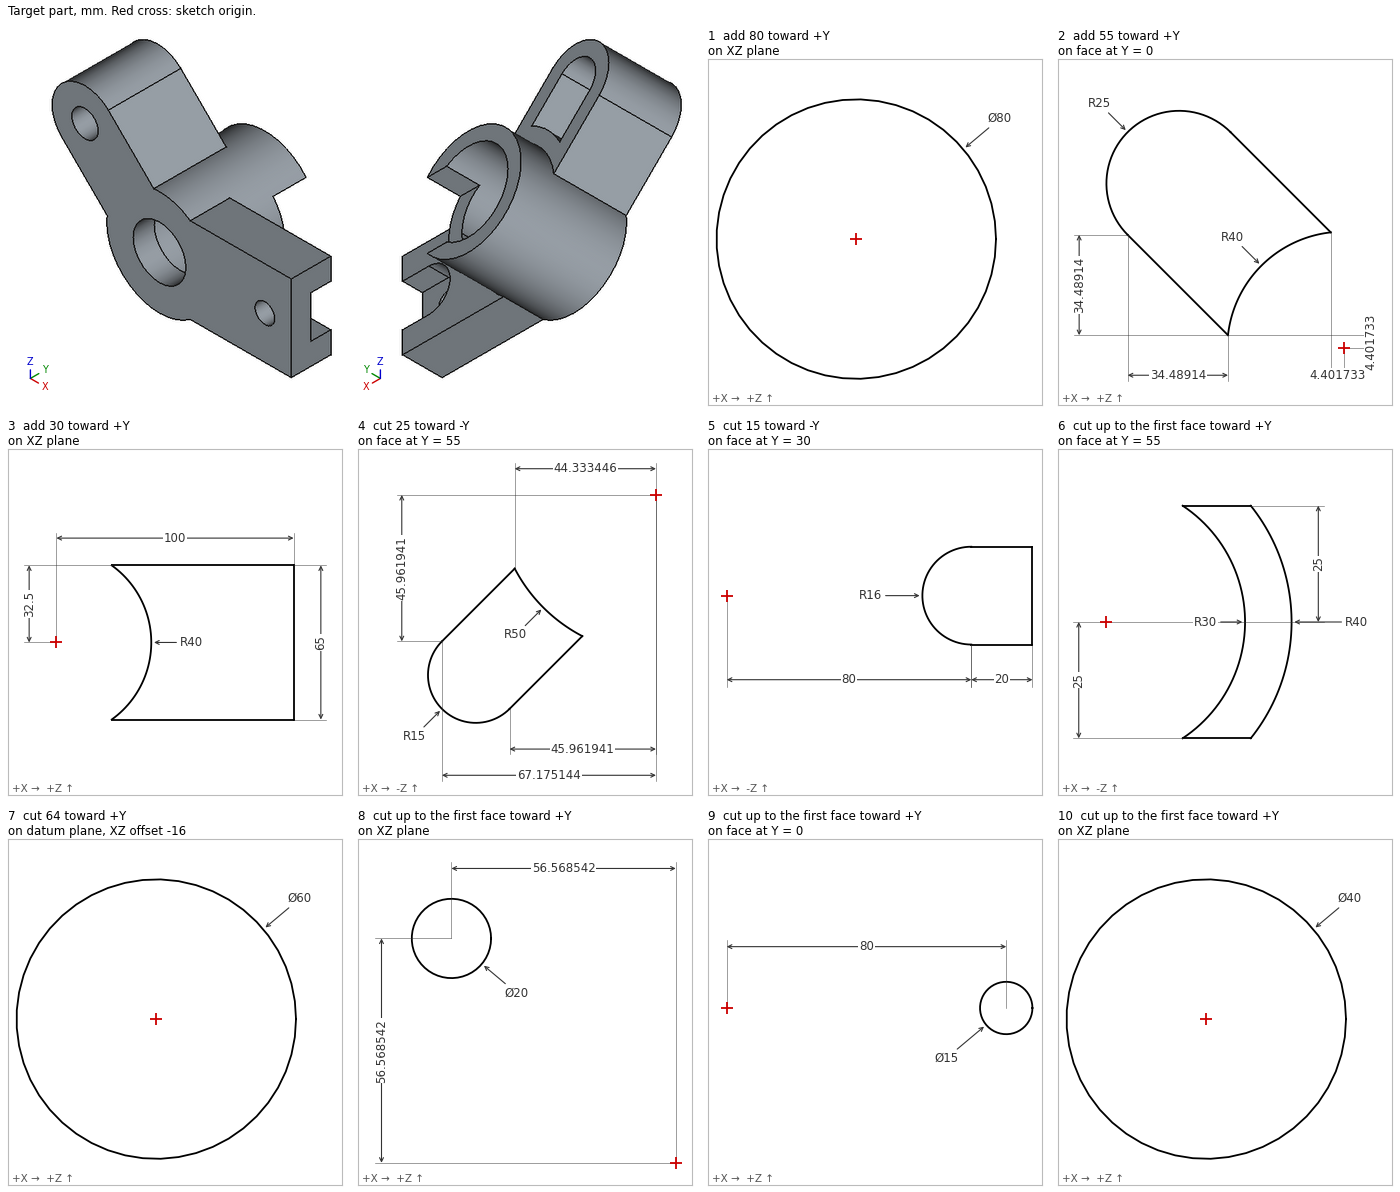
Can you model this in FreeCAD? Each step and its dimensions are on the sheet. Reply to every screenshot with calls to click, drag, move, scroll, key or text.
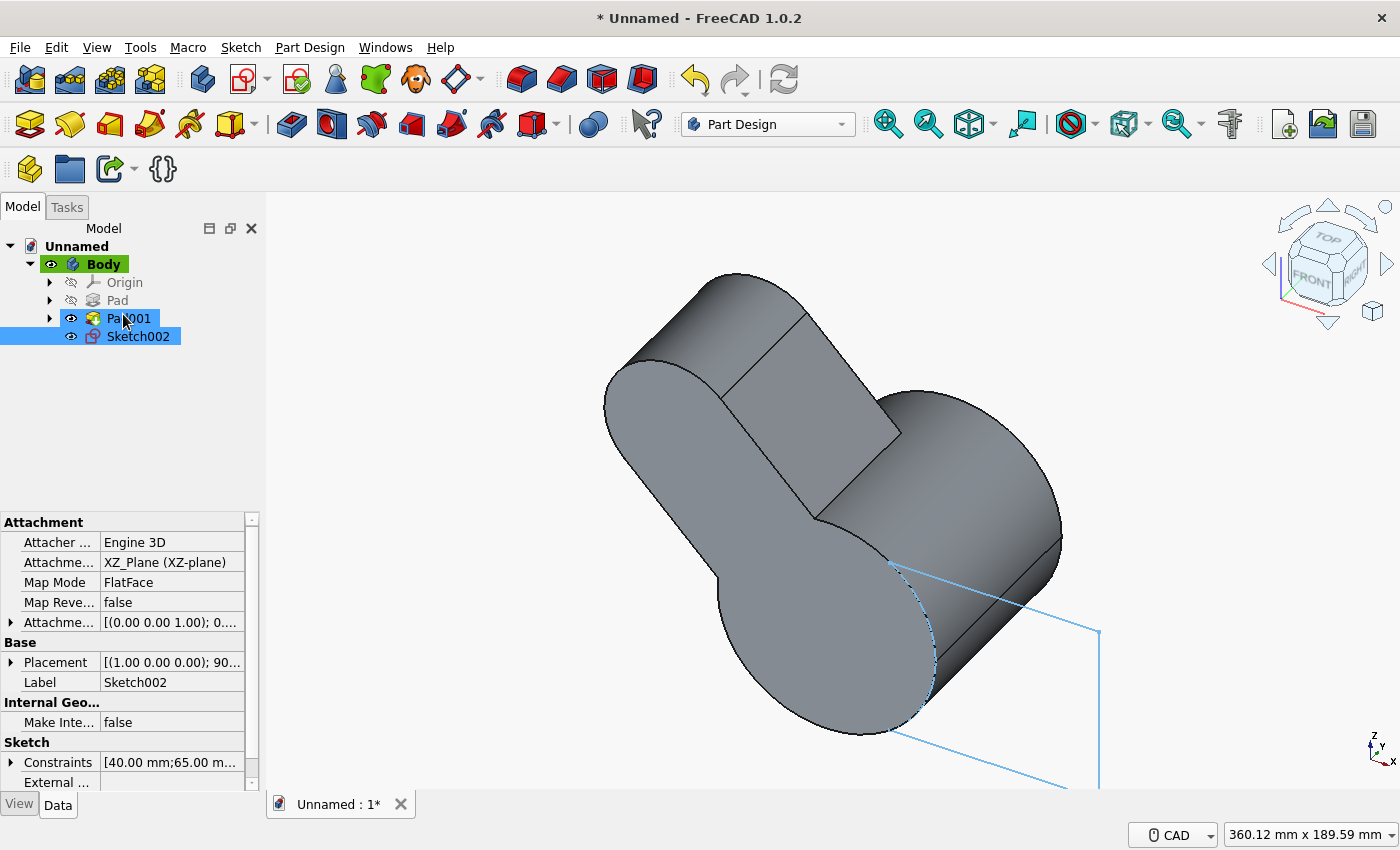
click(30, 124)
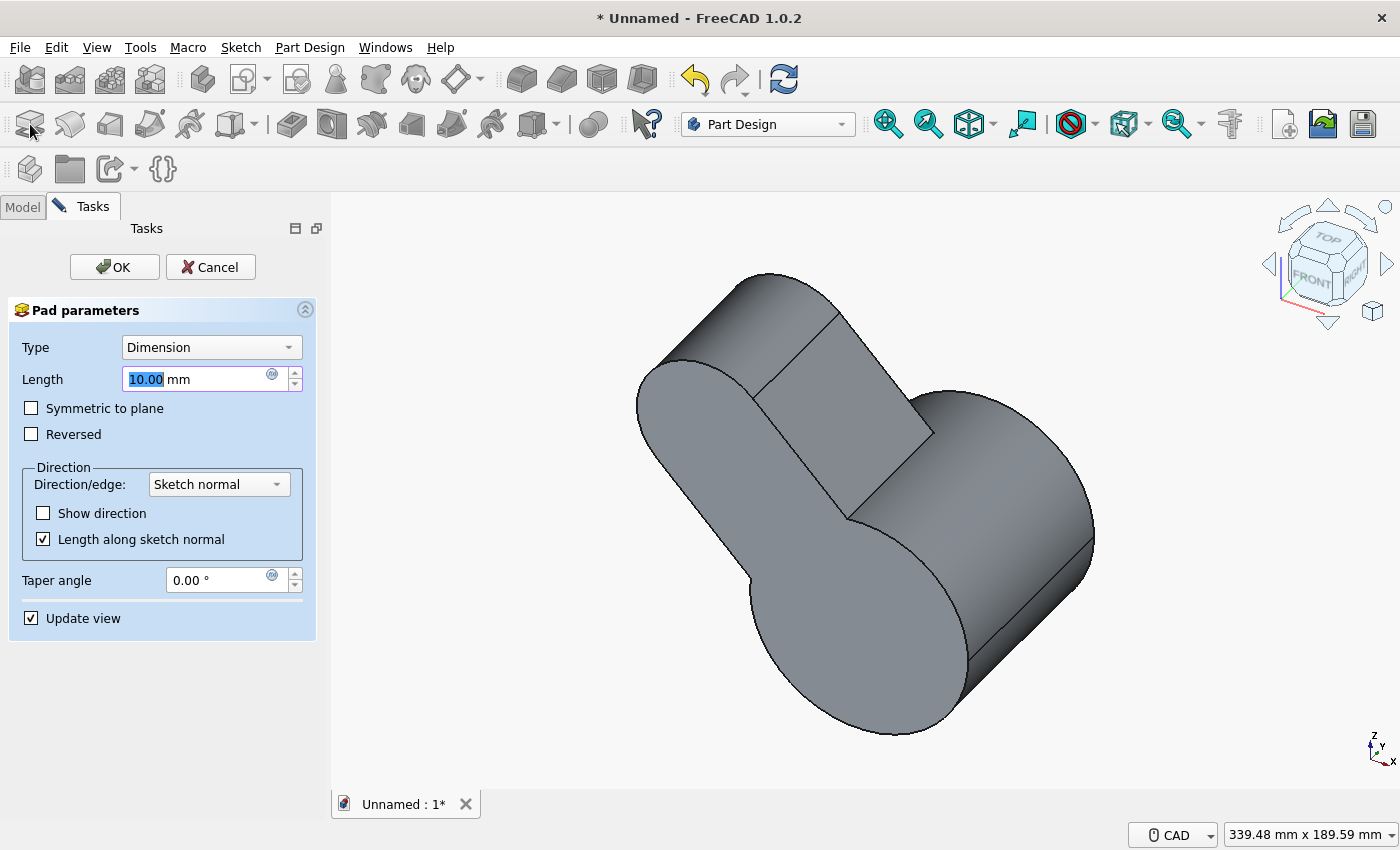
text(30)
key(Tab)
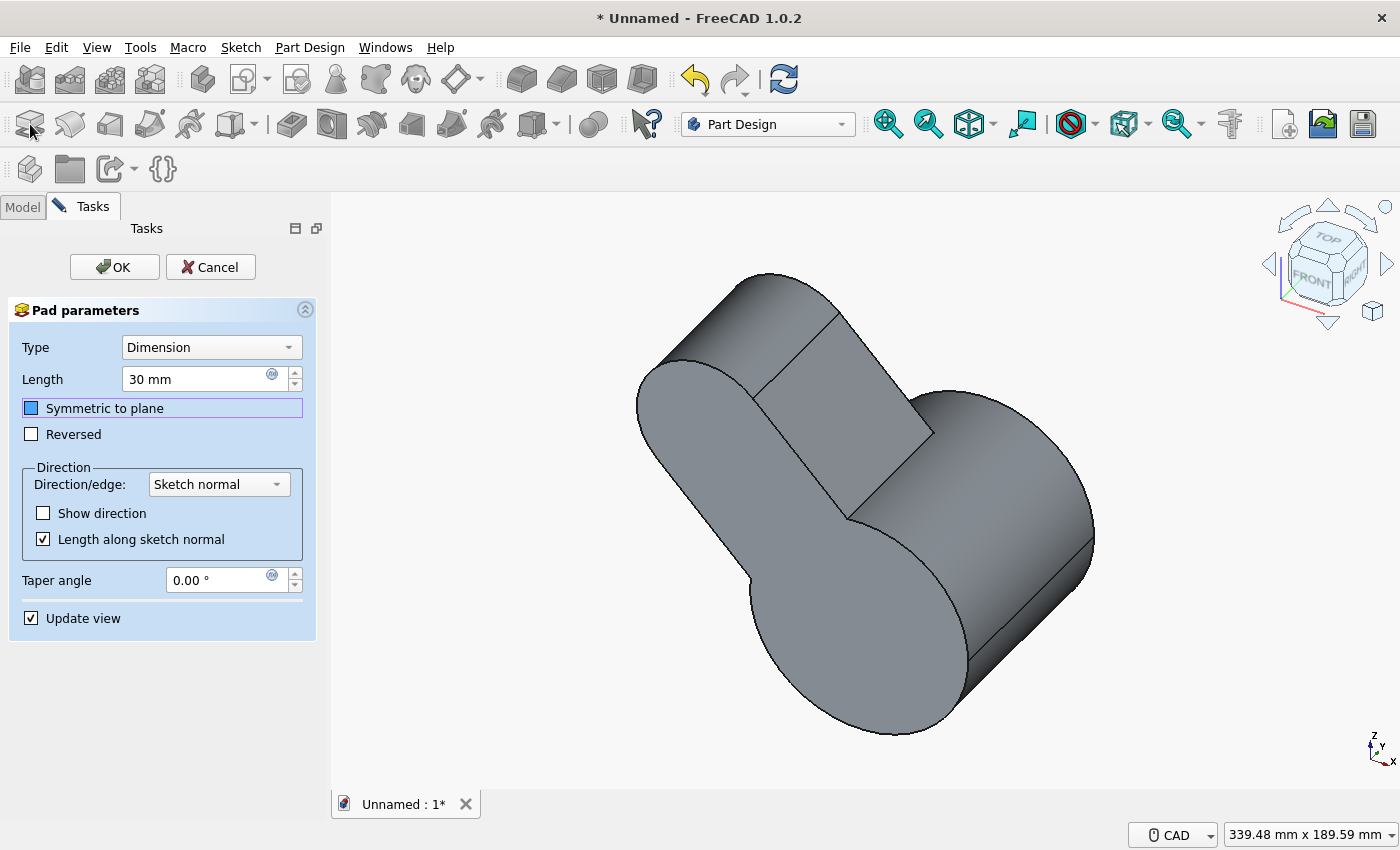
click(30, 434)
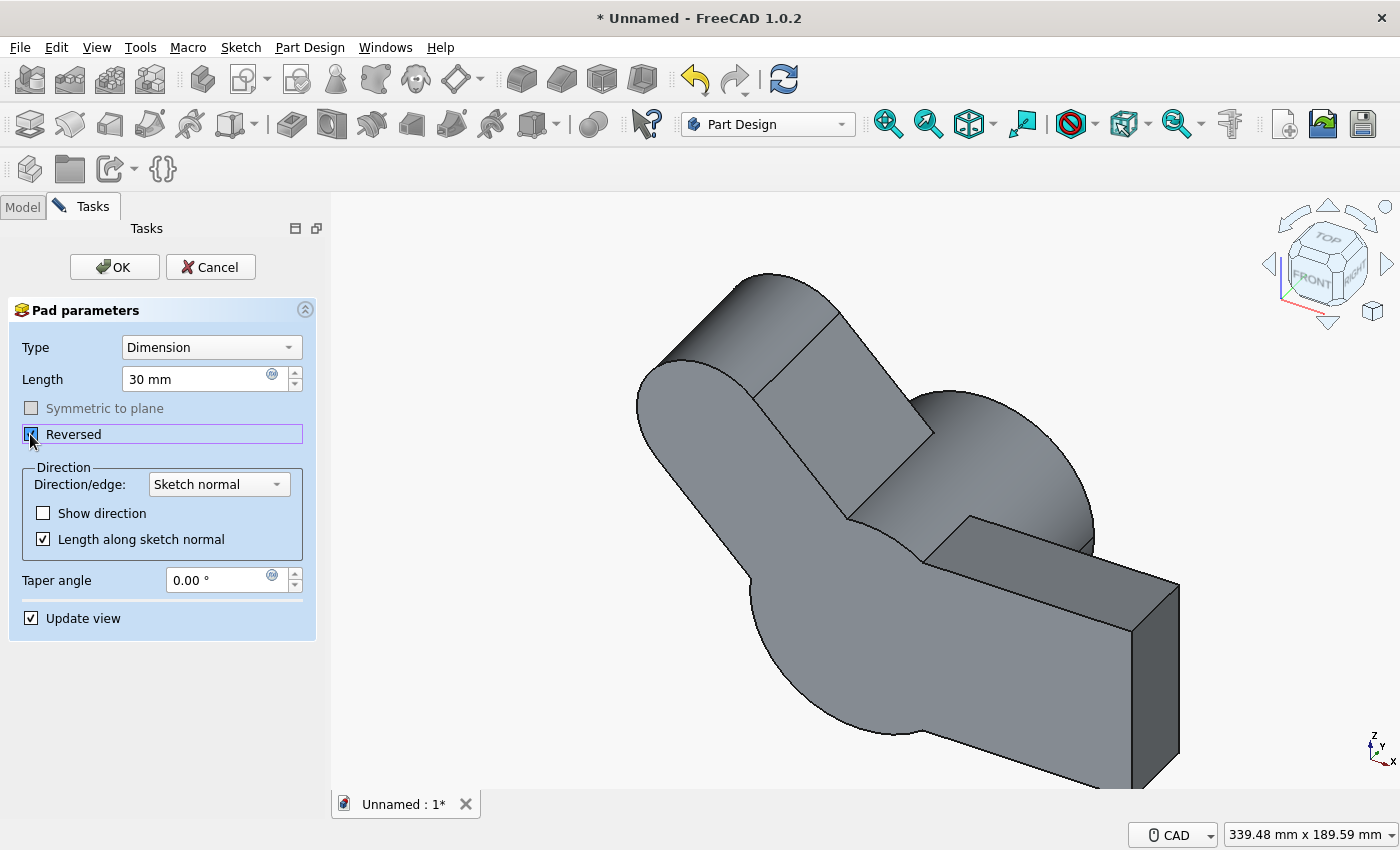
click(115, 267)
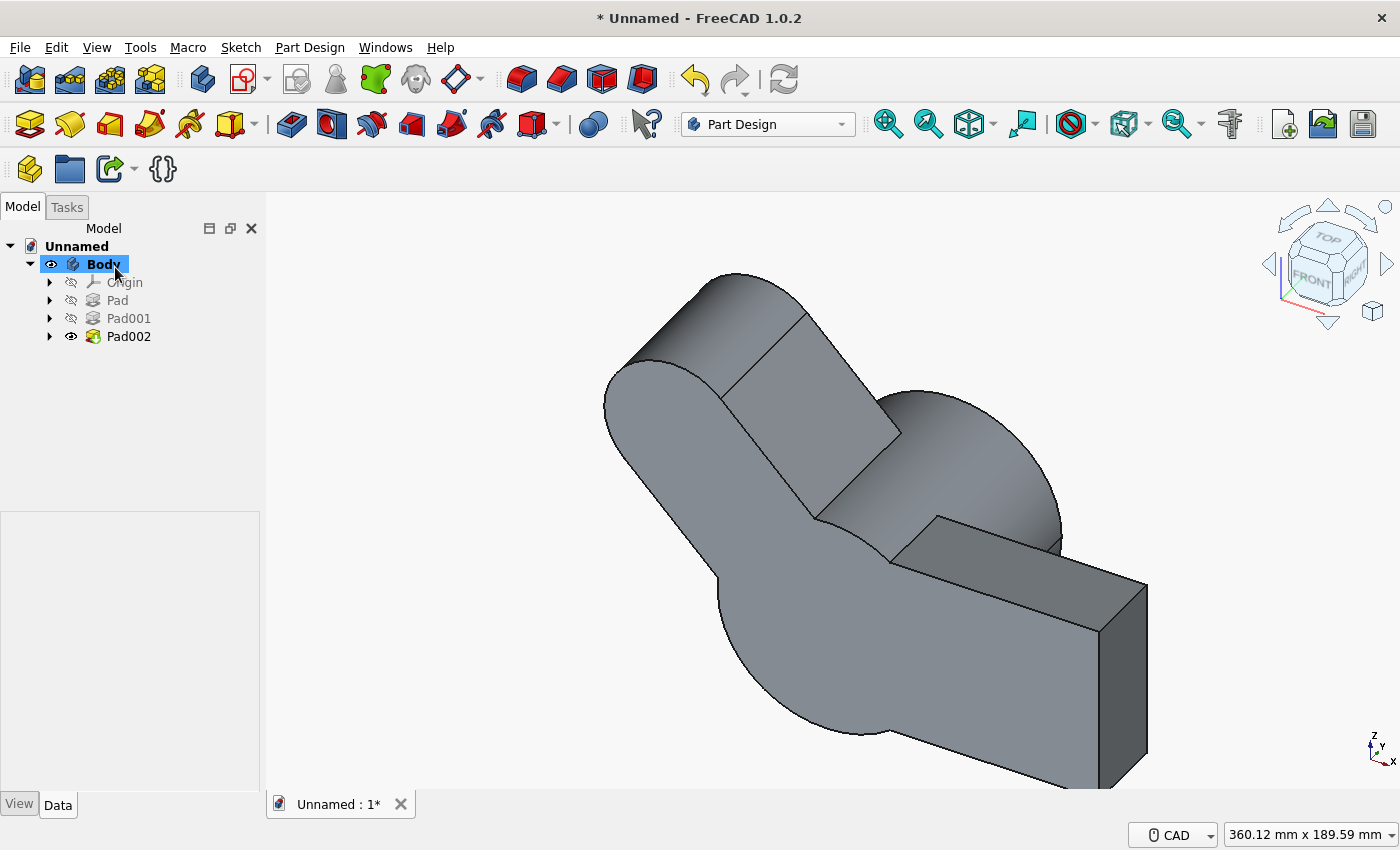
click(890, 124)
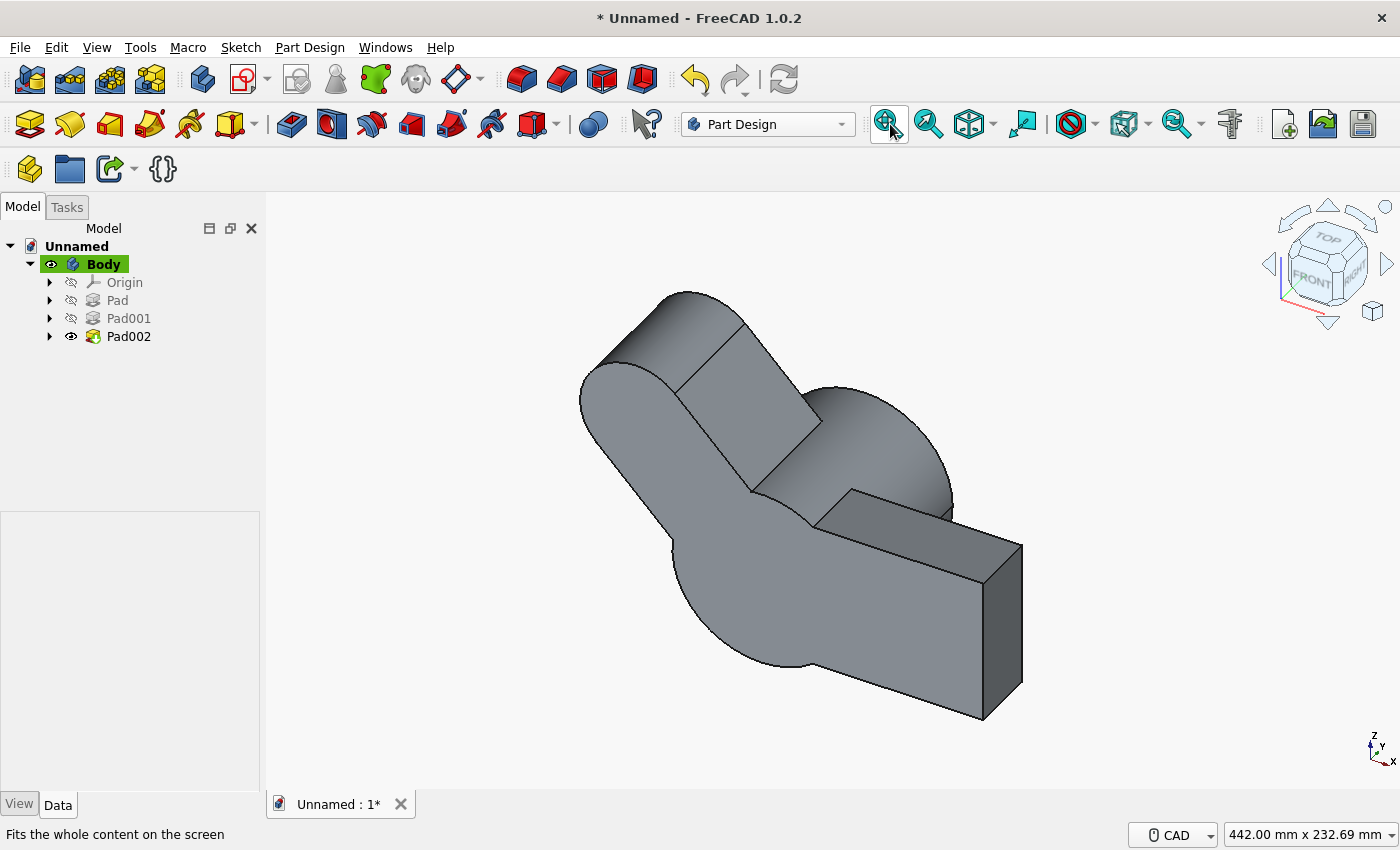
key(4)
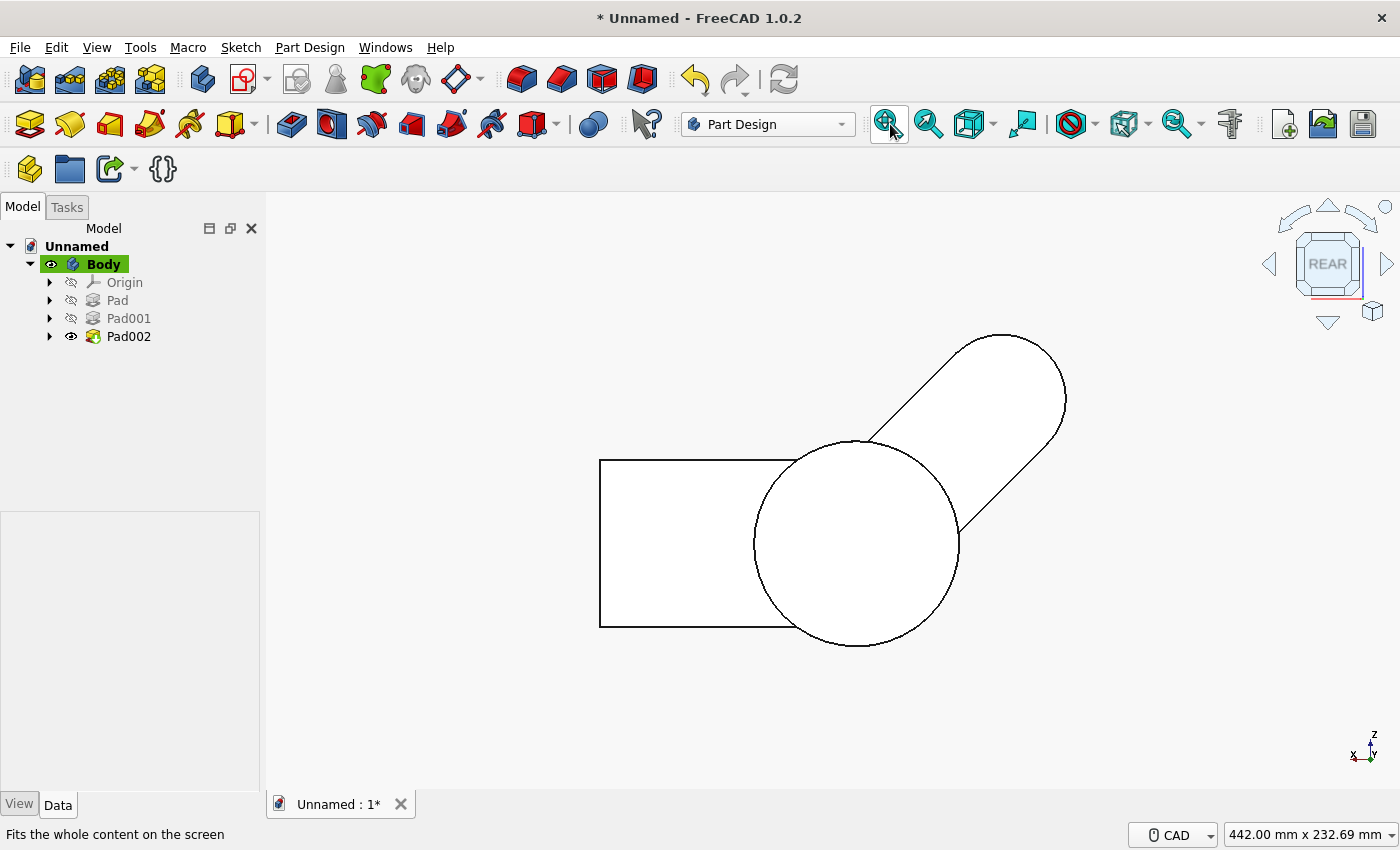
click(995, 404)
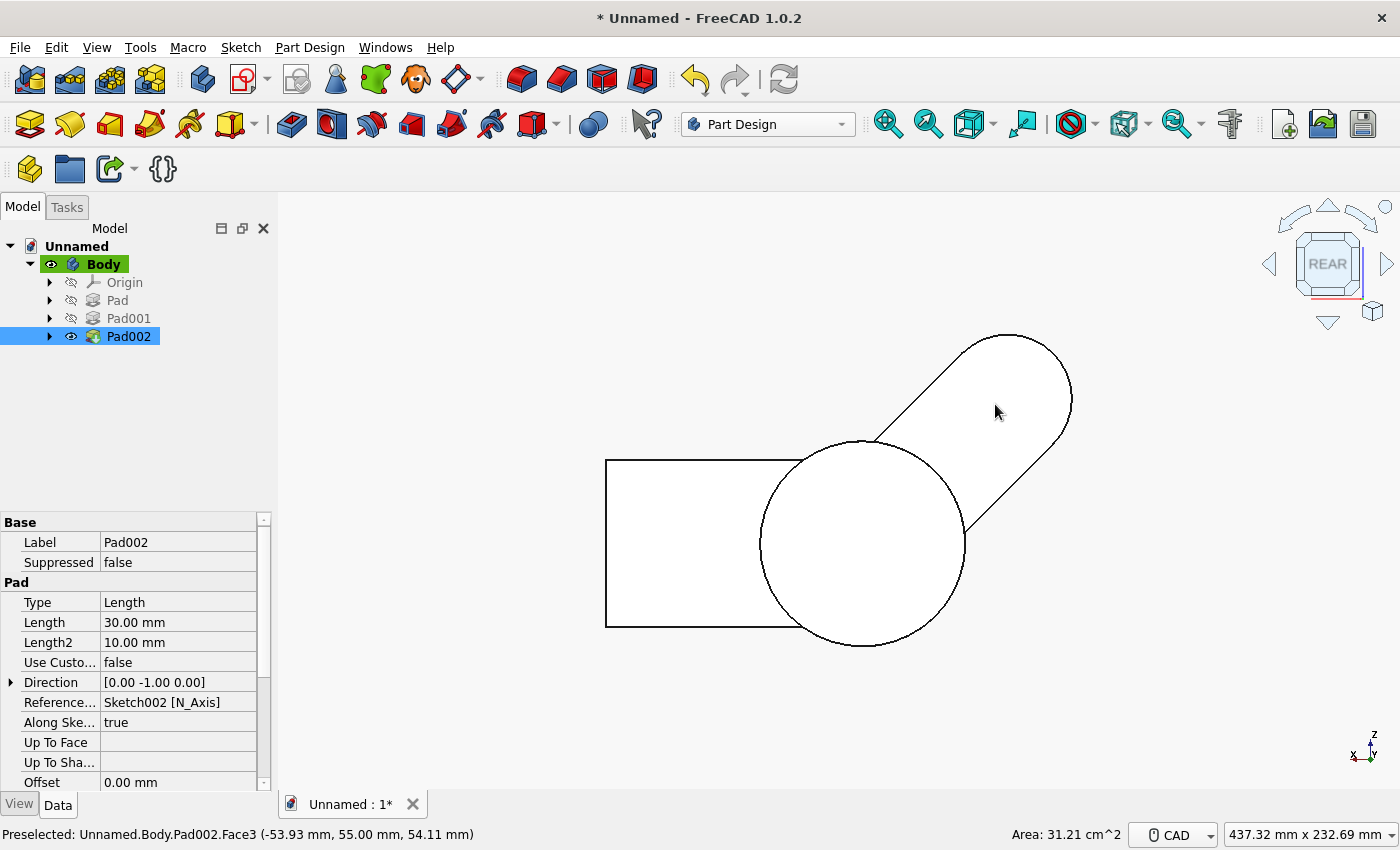
click(244, 80)